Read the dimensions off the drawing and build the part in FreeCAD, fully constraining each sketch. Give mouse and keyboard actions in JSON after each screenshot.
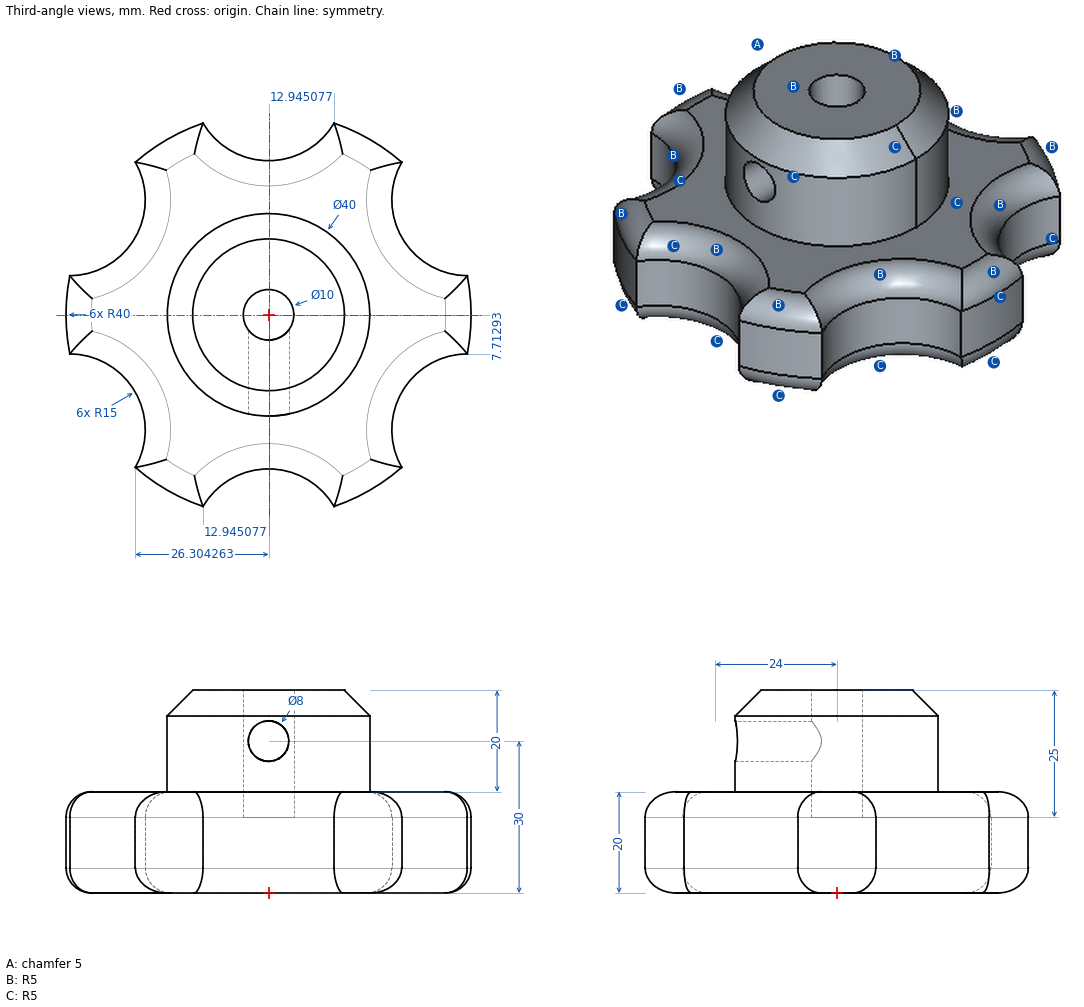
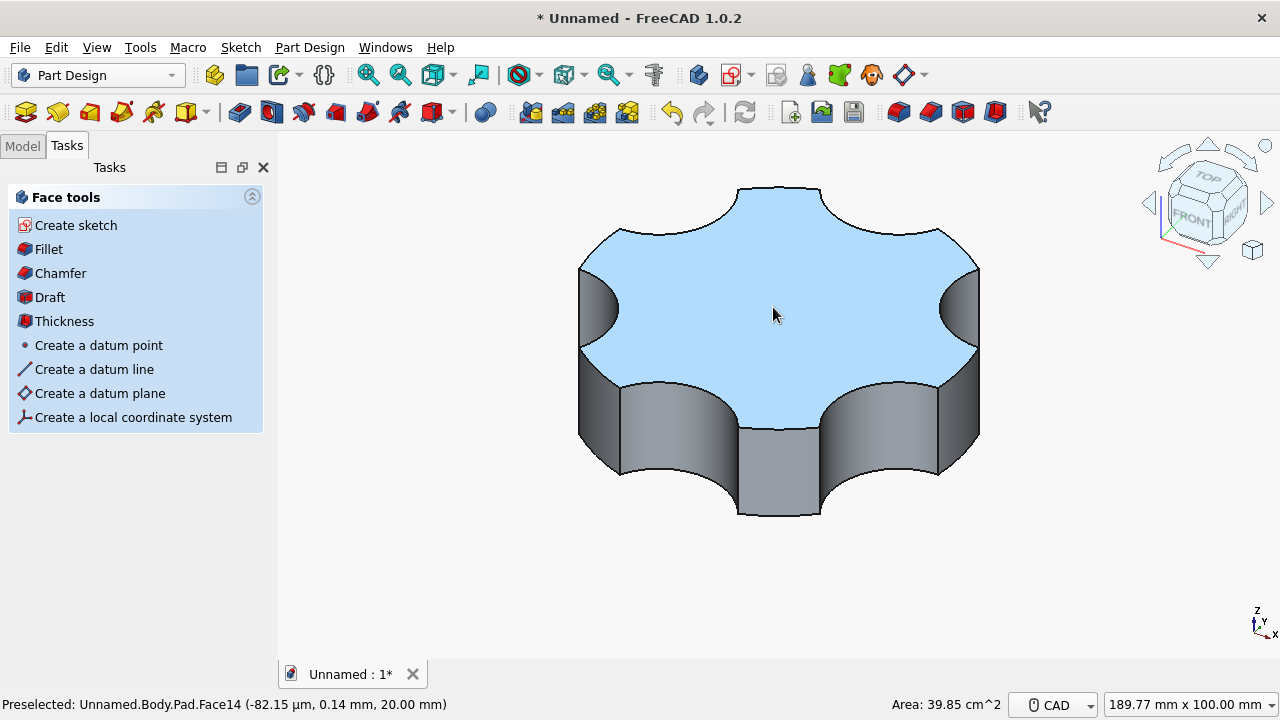
{"action": "left_click", "coordinate": [732, 76]}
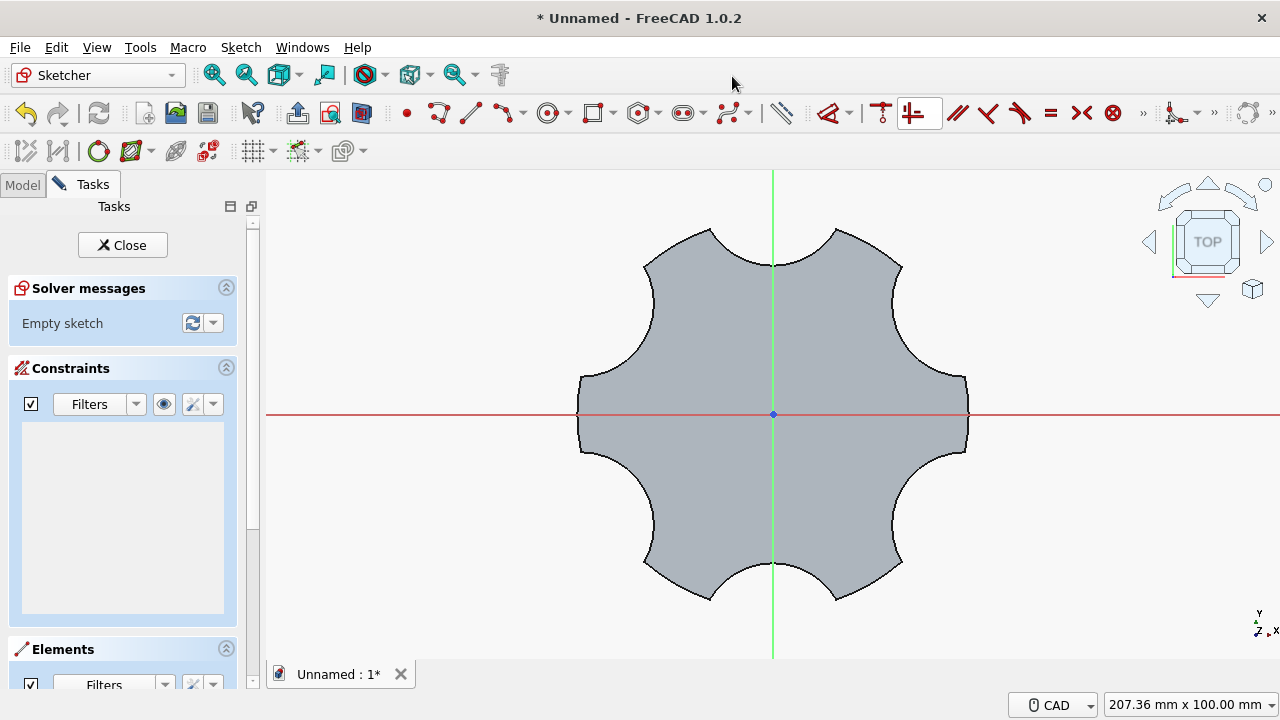
{"action": "scroll", "coordinate": [912, 414], "scroll_direction": "up", "scroll_amount": 2}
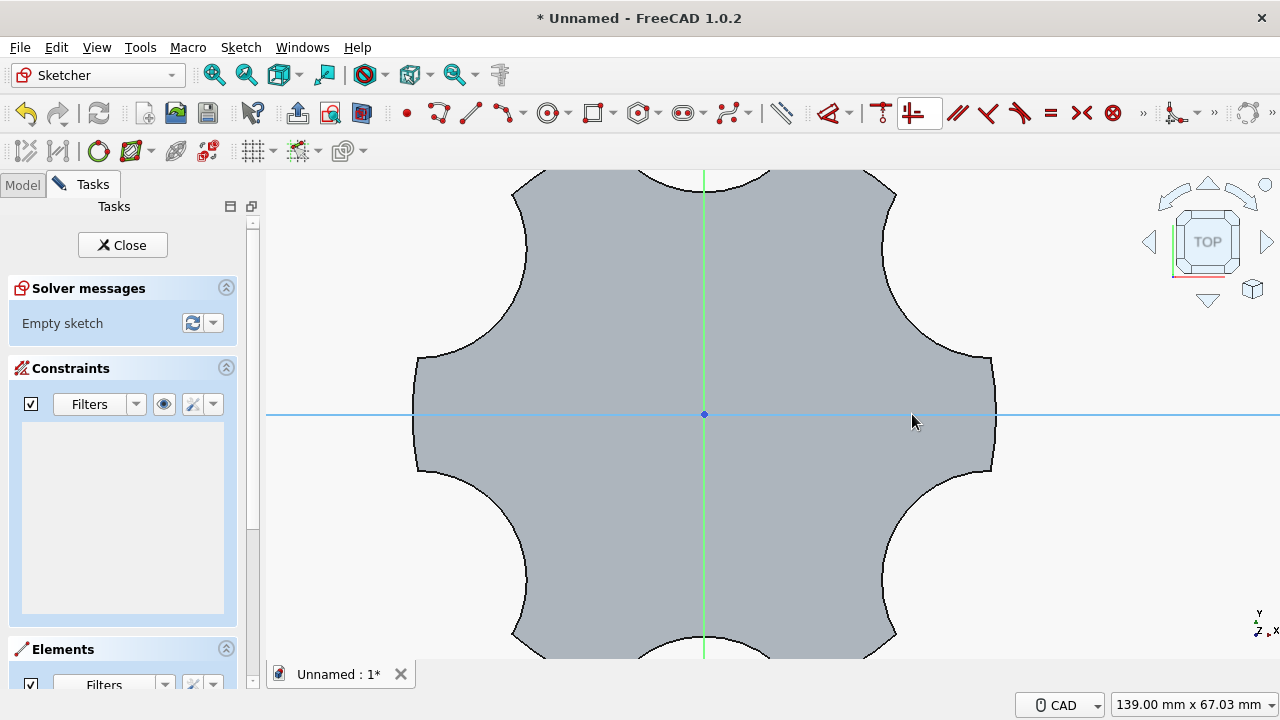
{"action": "left_click", "coordinate": [548, 114]}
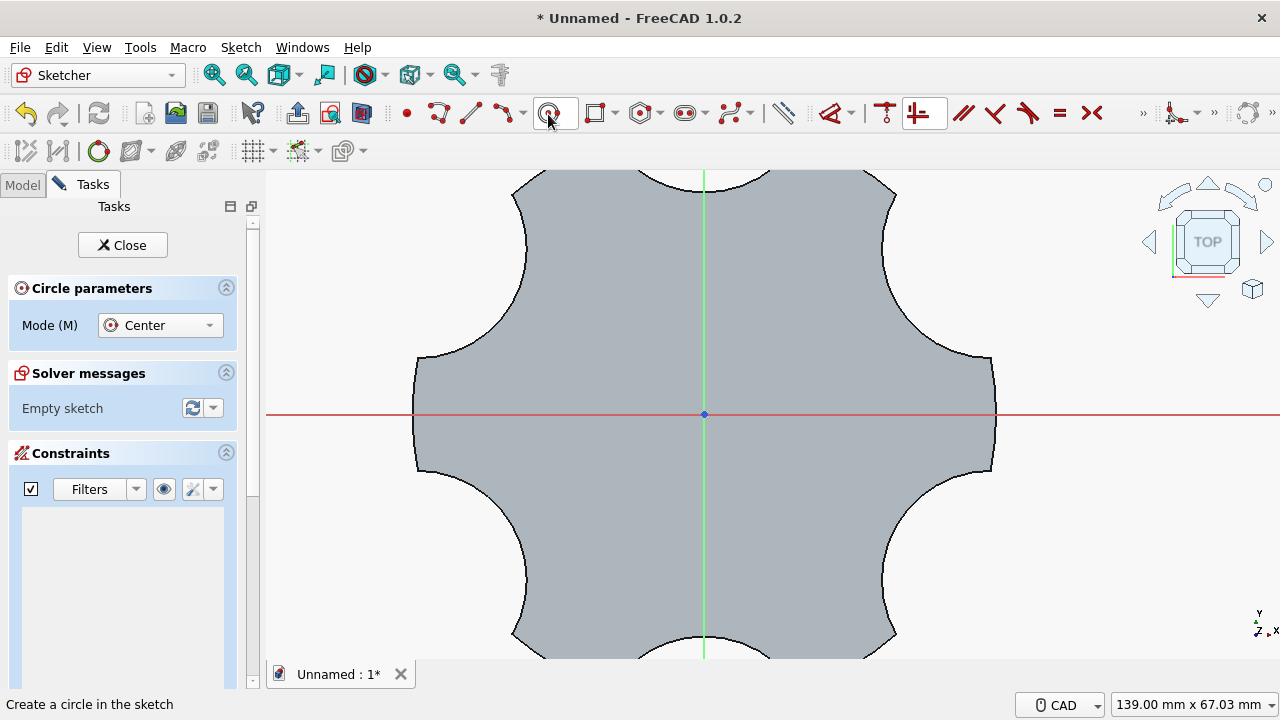
{"action": "left_click", "coordinate": [704, 414]}
{"action": "mouse_move", "coordinate": [807, 311]}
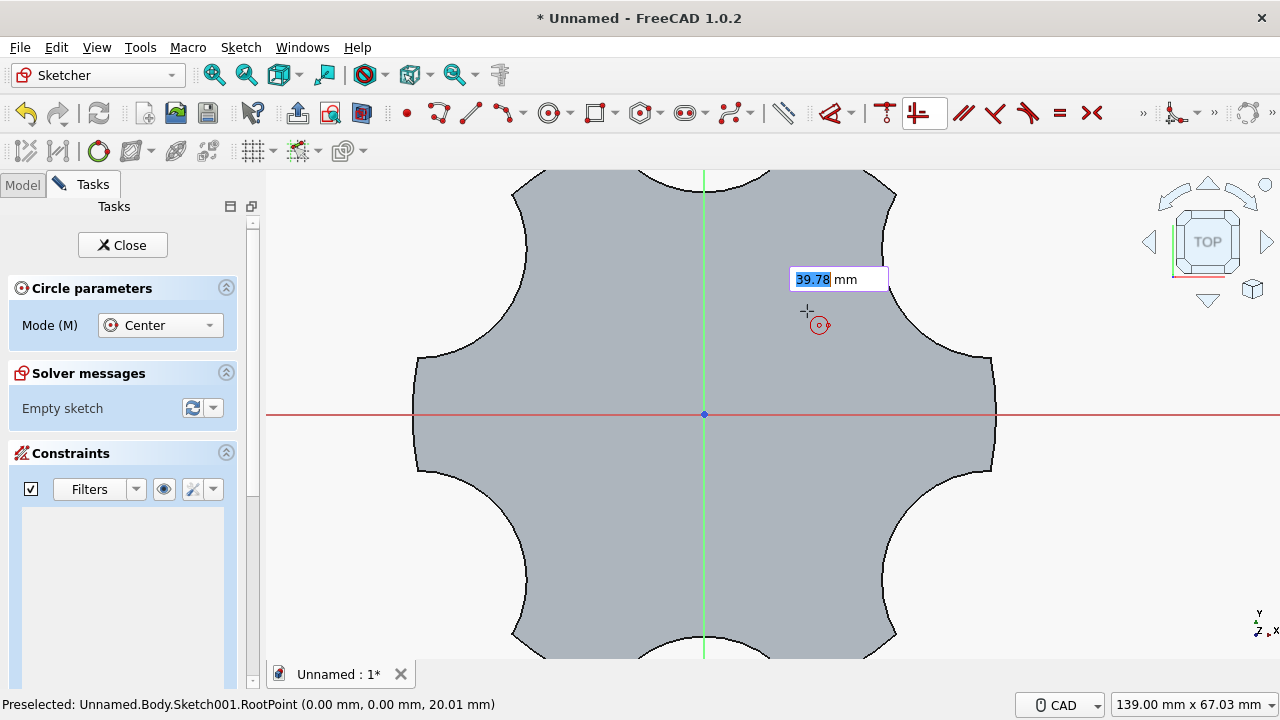
{"action": "type", "text": "40"}
{"action": "key", "text": "Return"}
{"action": "key", "text": "Escape"}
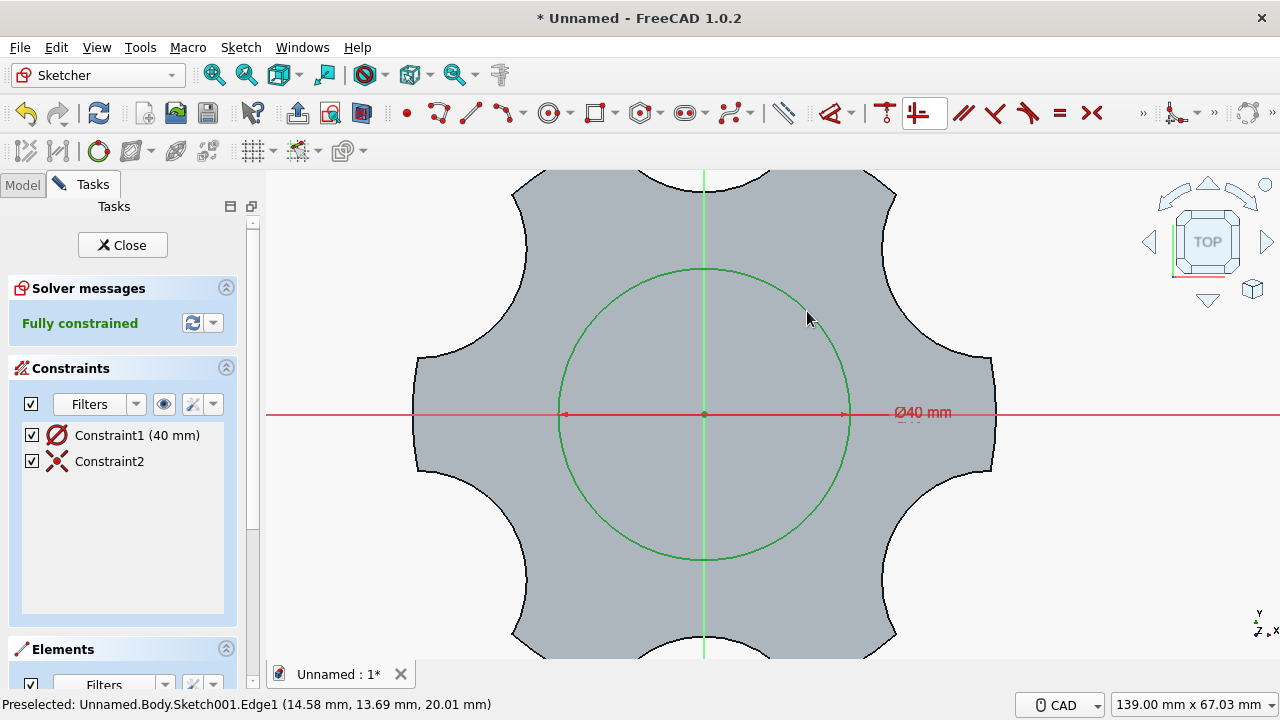
{"action": "left_click", "coordinate": [123, 245]}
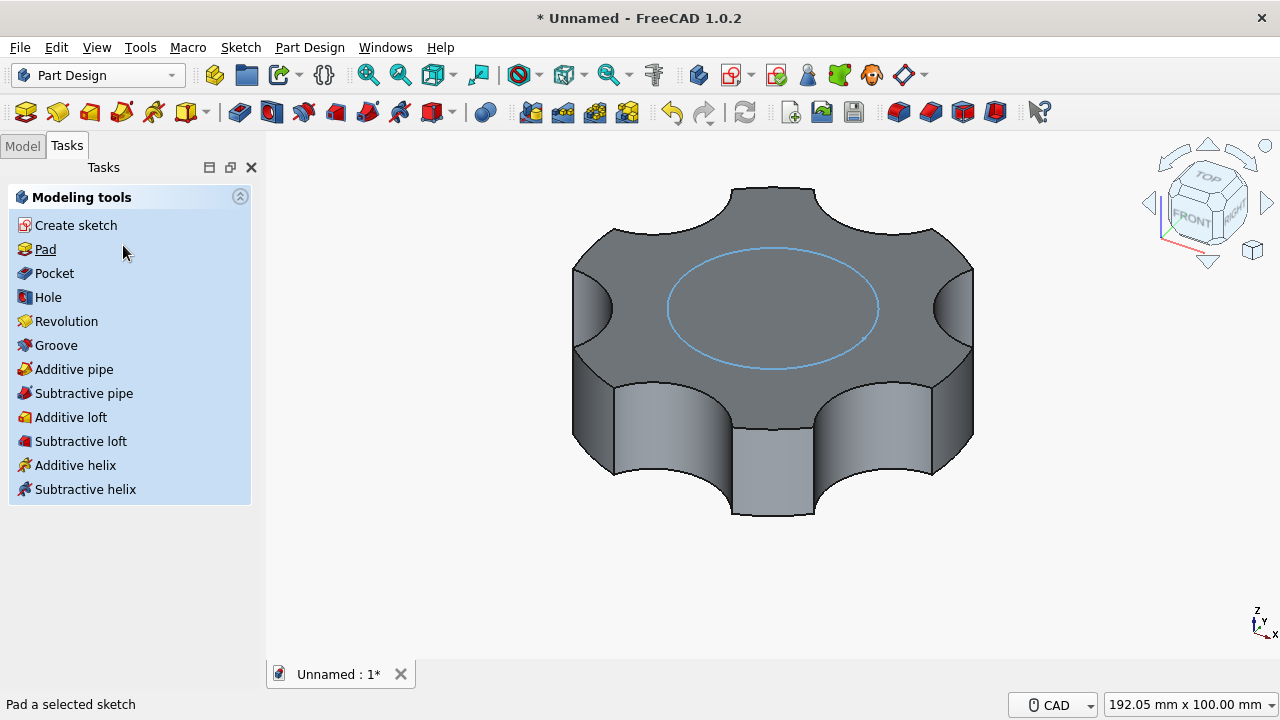
{"action": "left_click", "coordinate": [26, 112]}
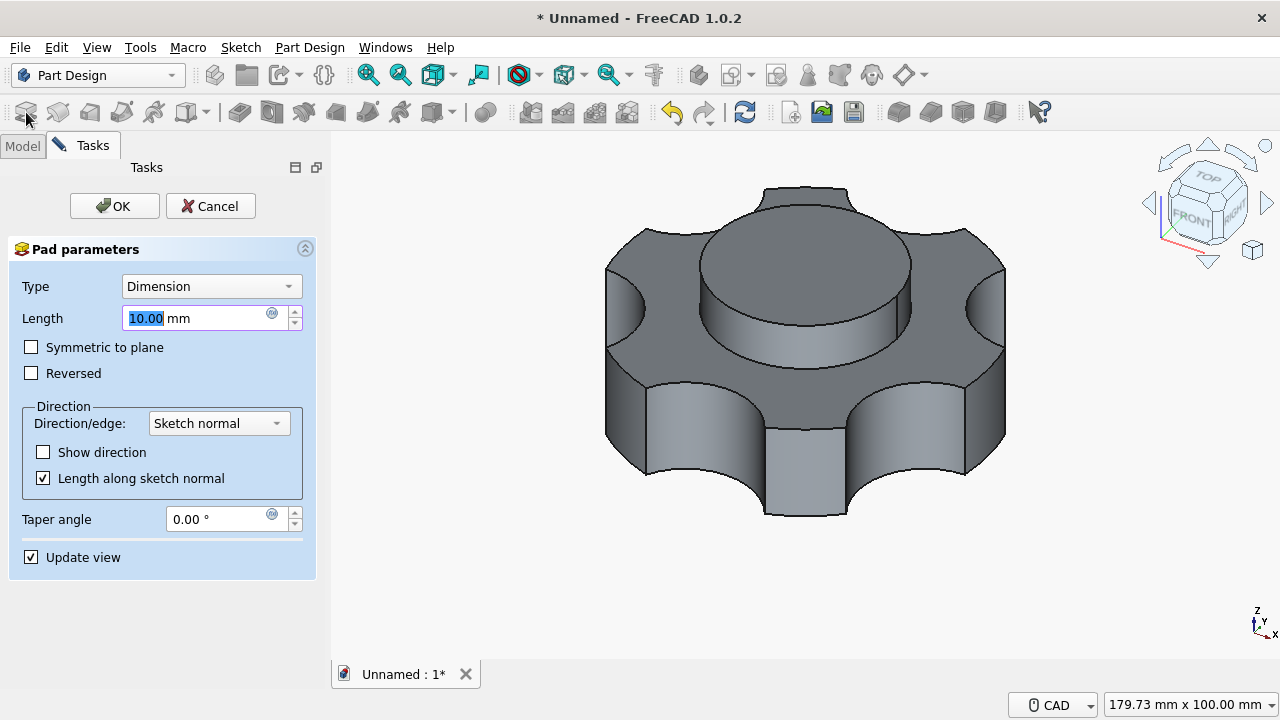
{"action": "type", "text": "20"}
{"action": "key", "text": "Tab"}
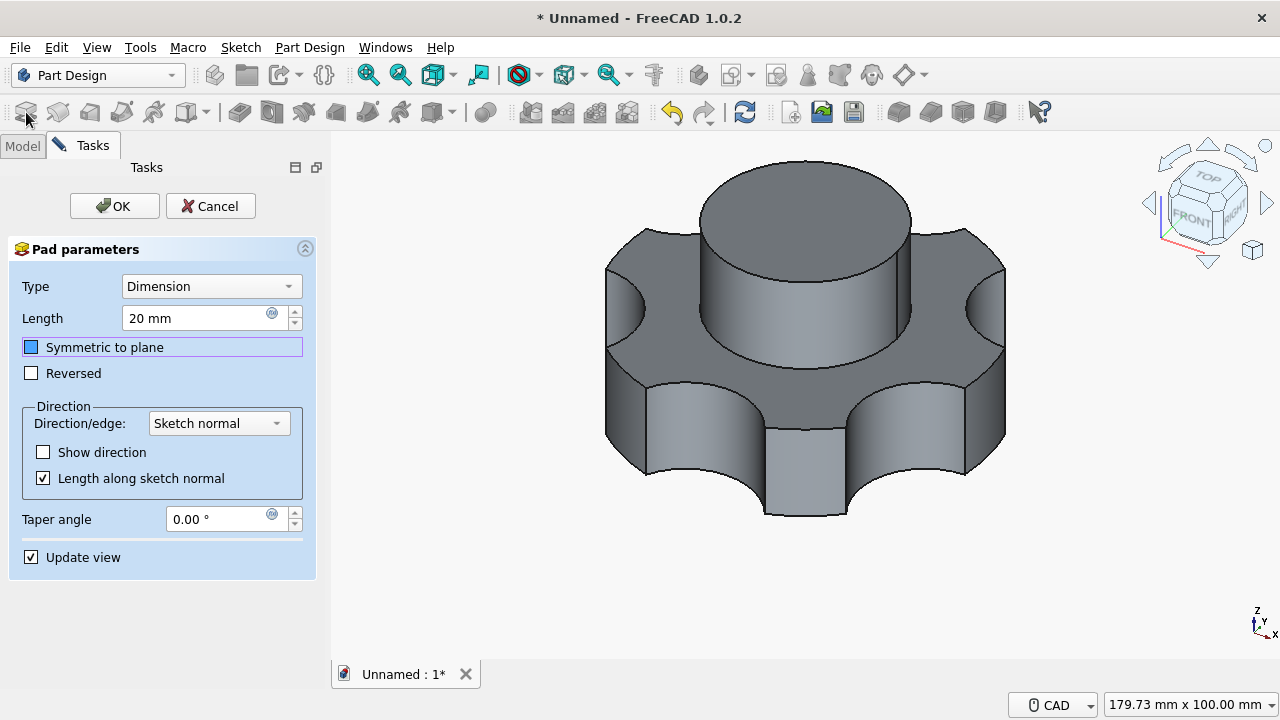
{"action": "left_click", "coordinate": [115, 206]}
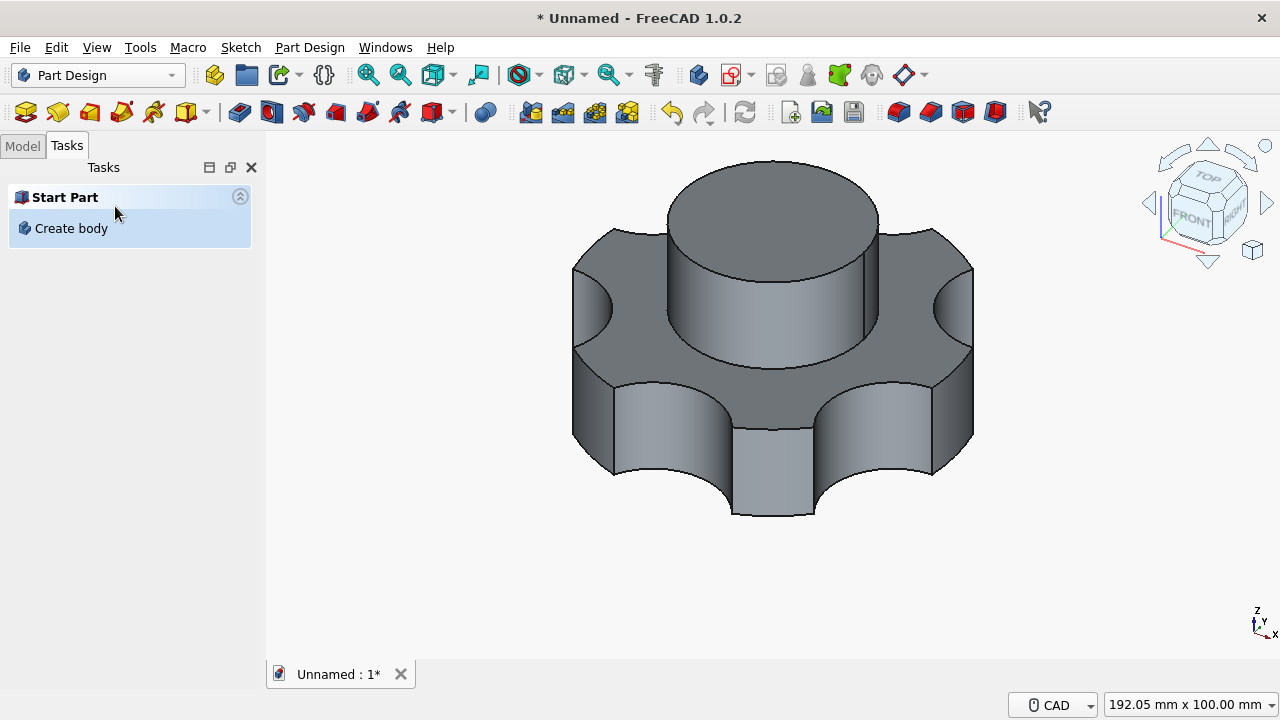
{"action": "left_click", "coordinate": [370, 76]}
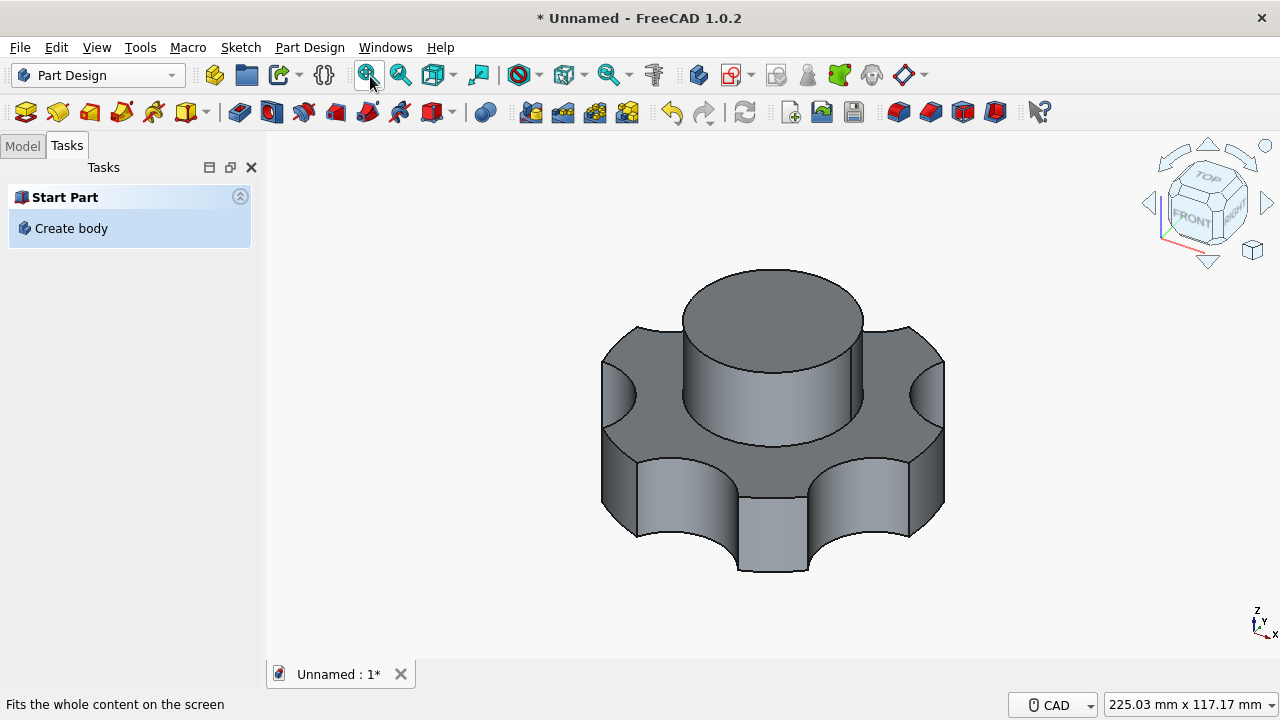
{"action": "left_click", "coordinate": [773, 320]}